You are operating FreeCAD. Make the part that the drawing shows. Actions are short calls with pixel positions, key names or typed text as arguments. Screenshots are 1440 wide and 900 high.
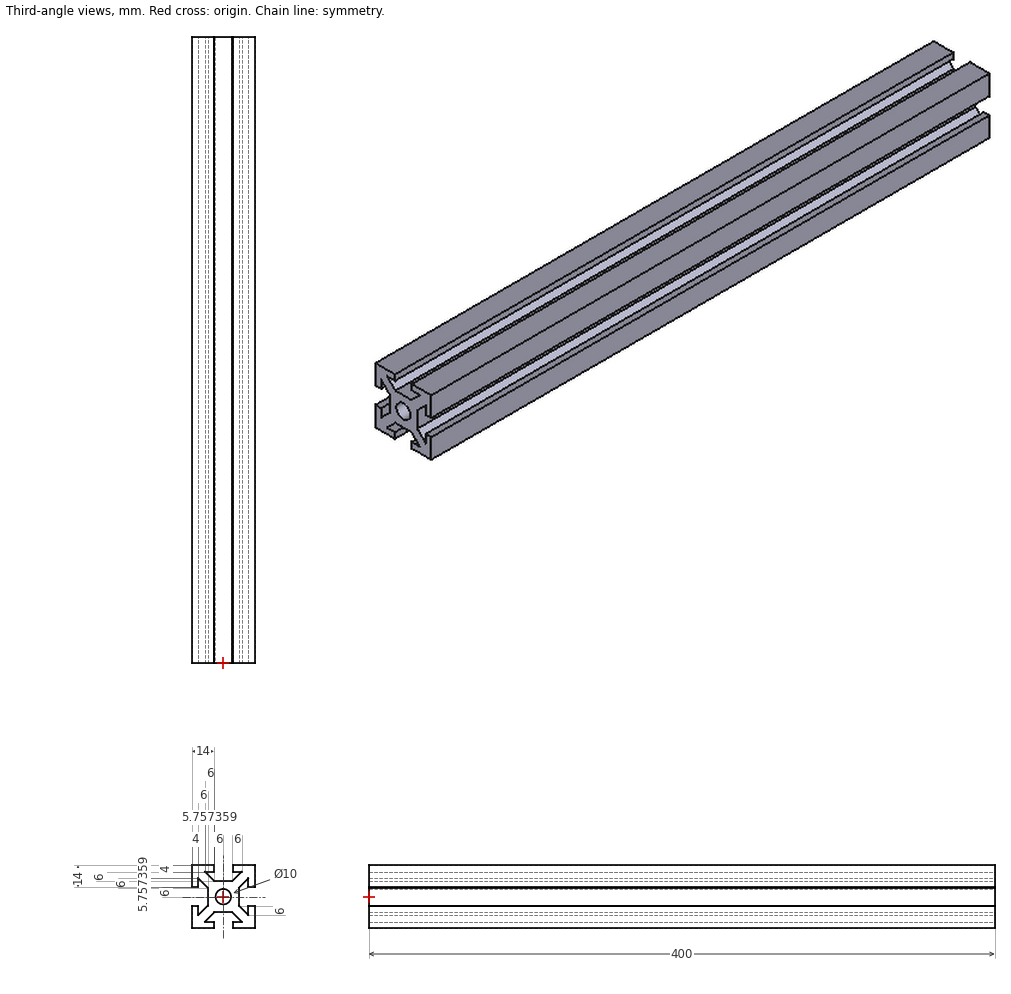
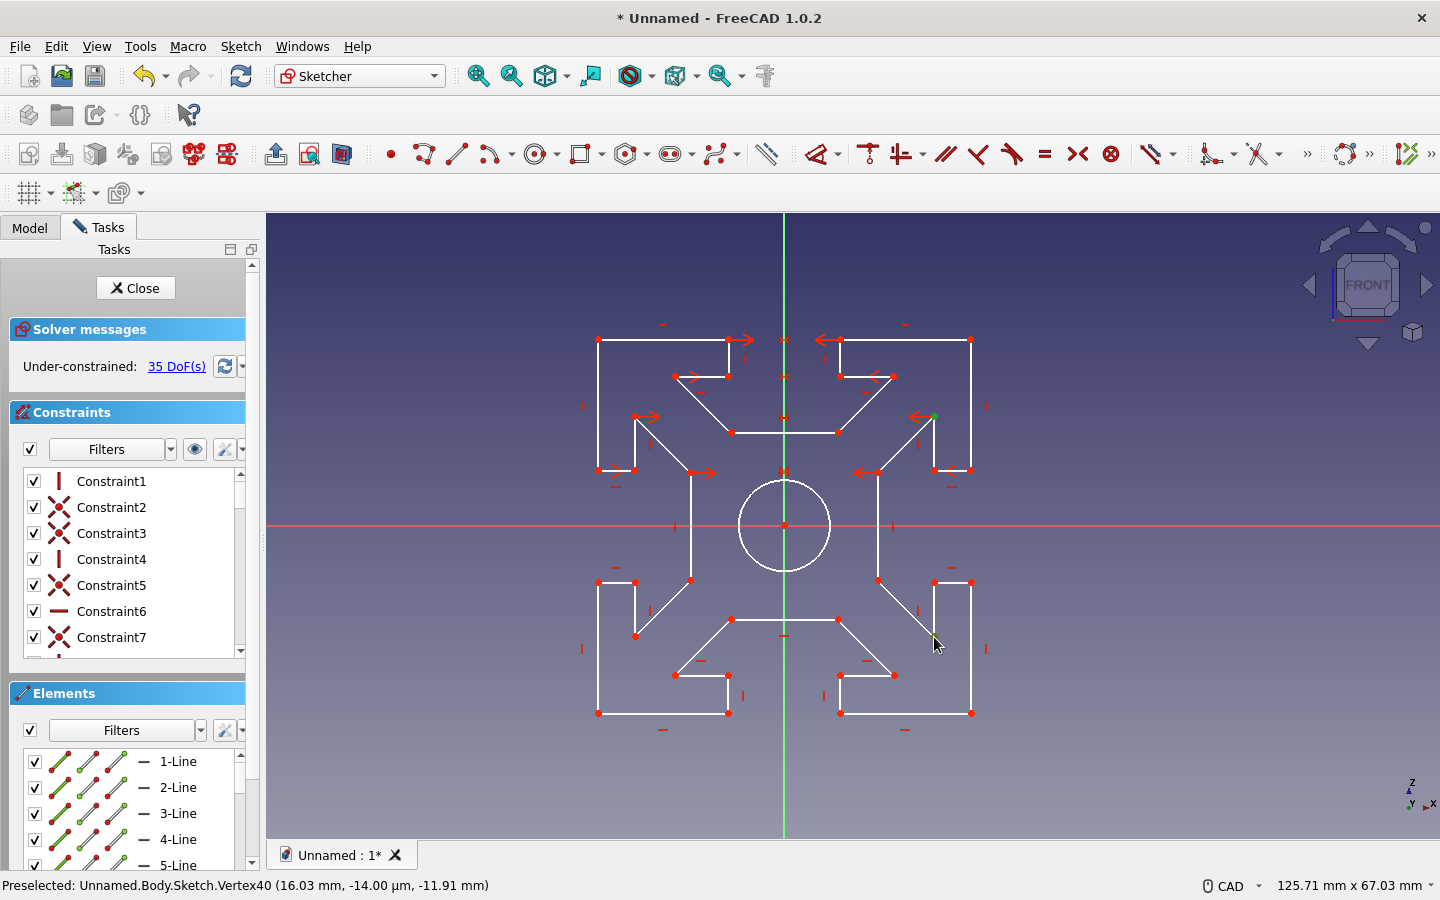
click(364, 526)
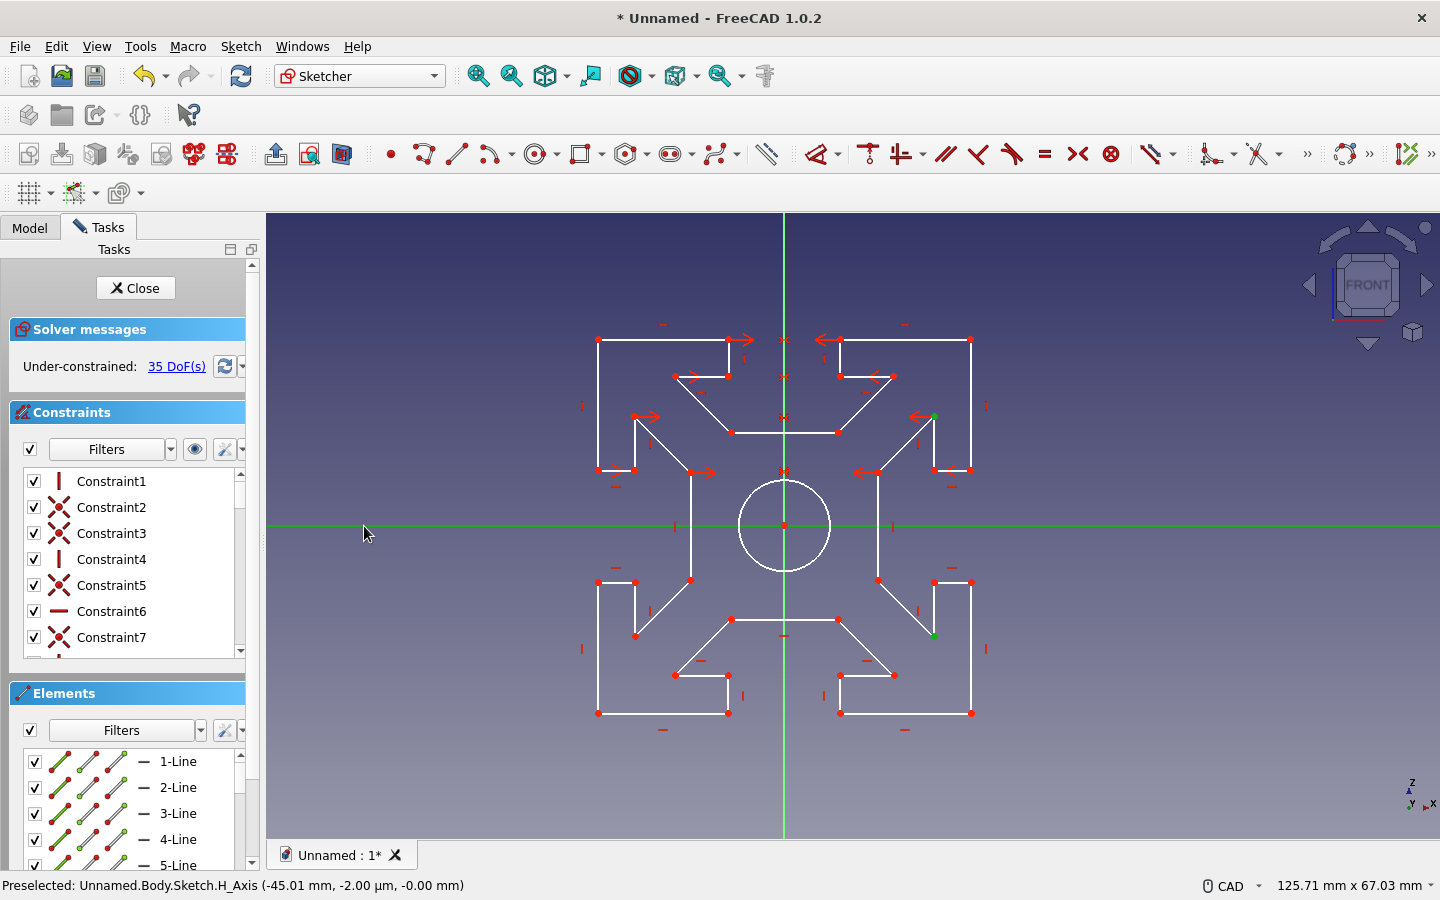
key(s)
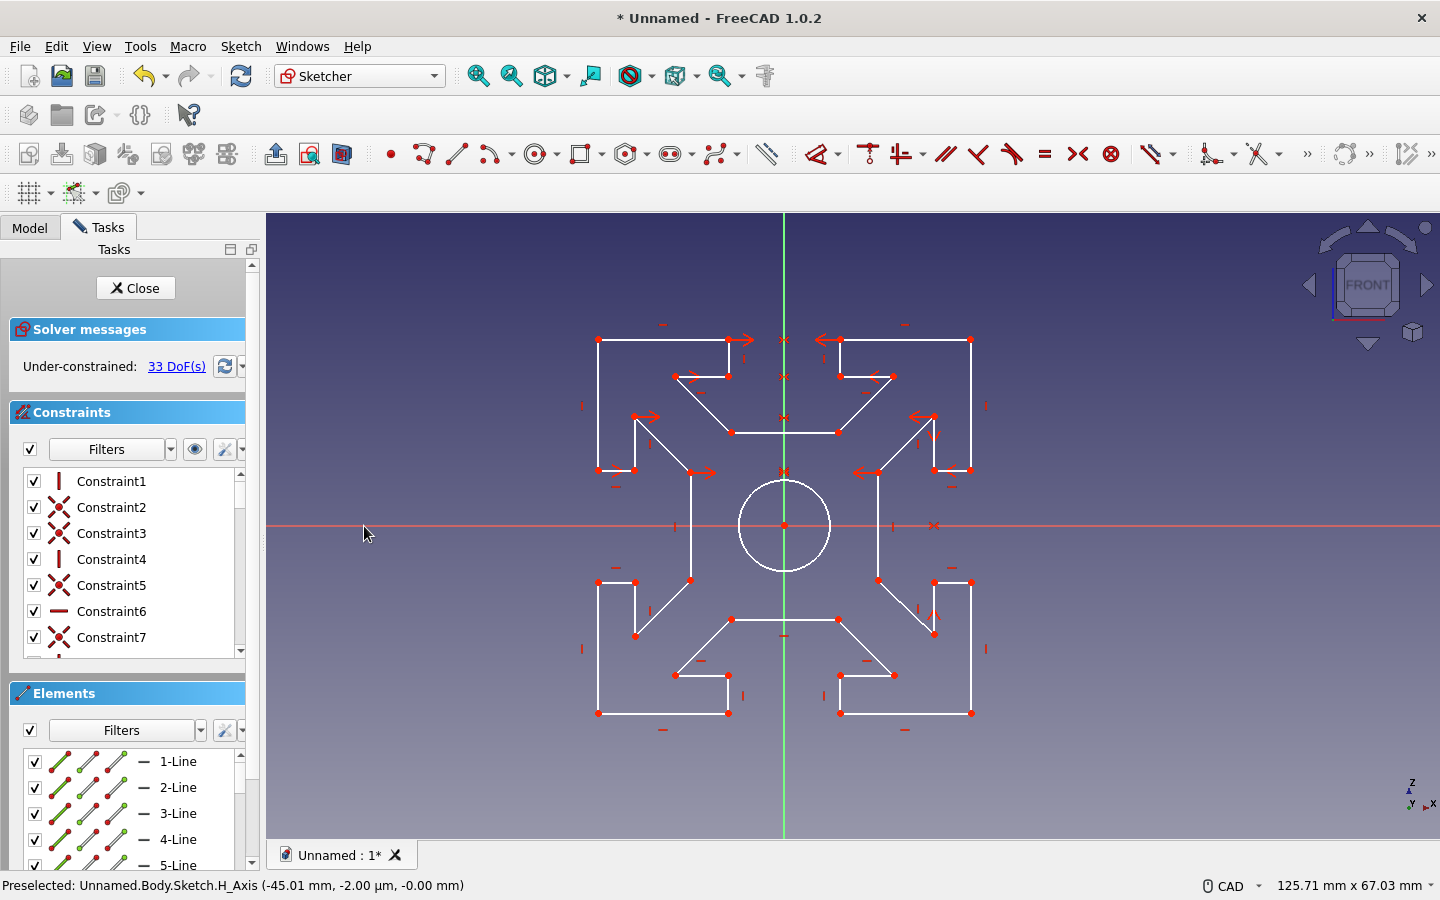
click(971, 471)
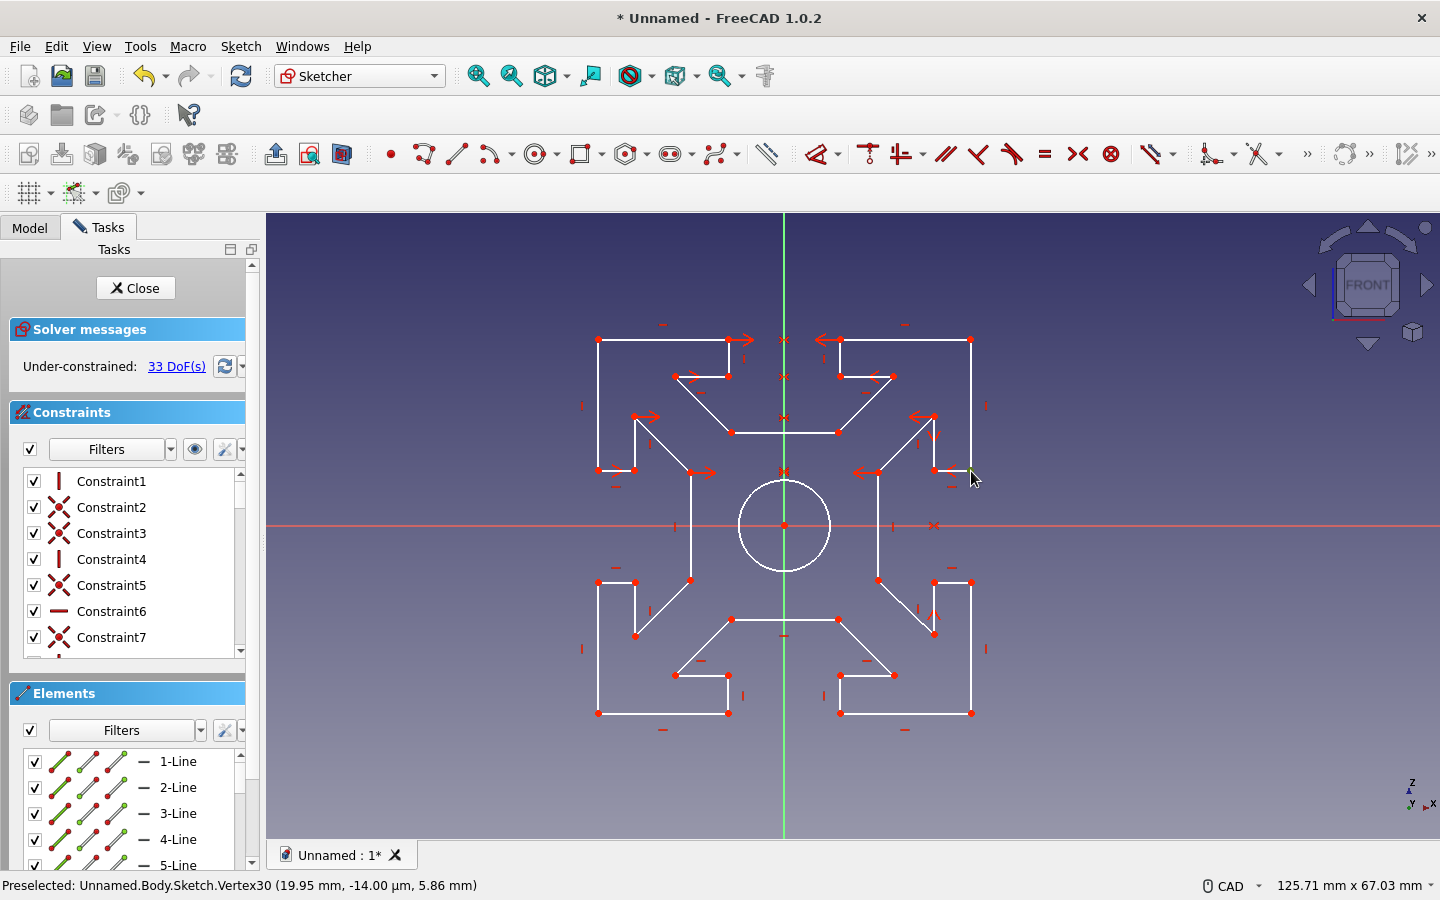
click(971, 583)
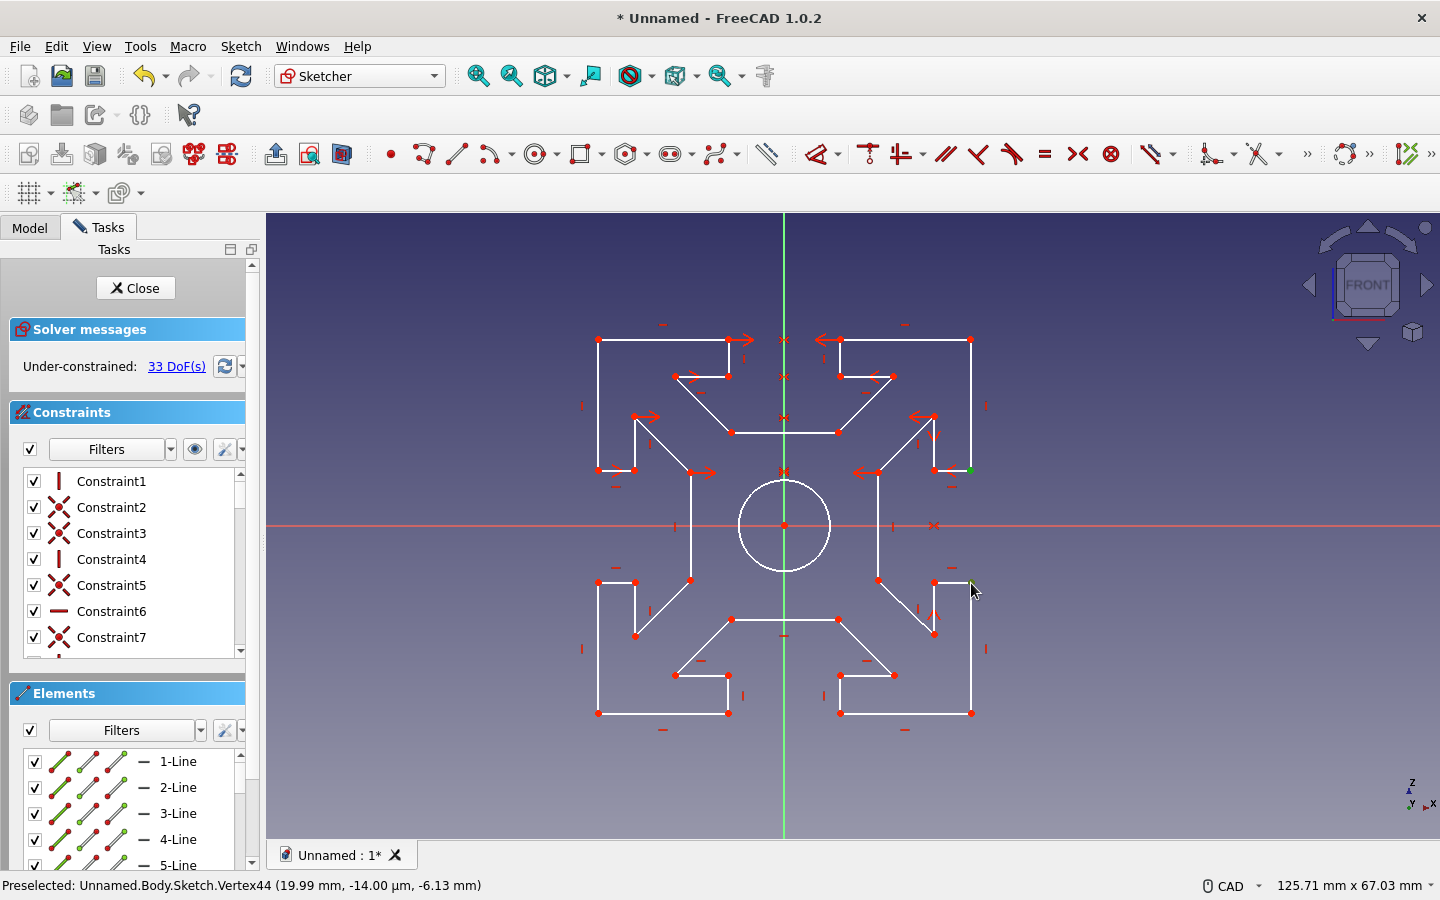
click(364, 526)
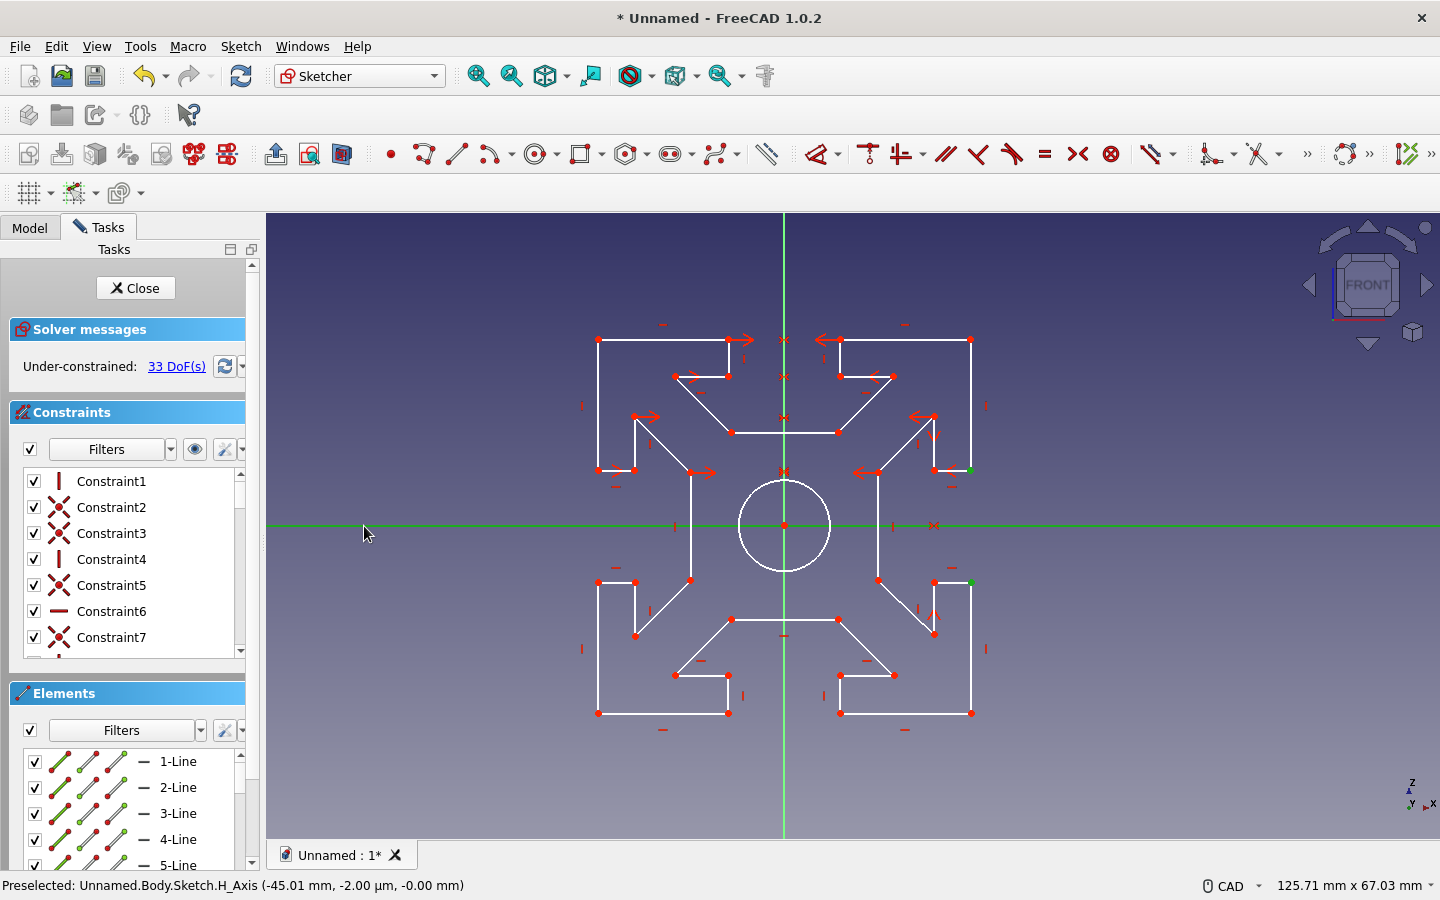
click(1078, 154)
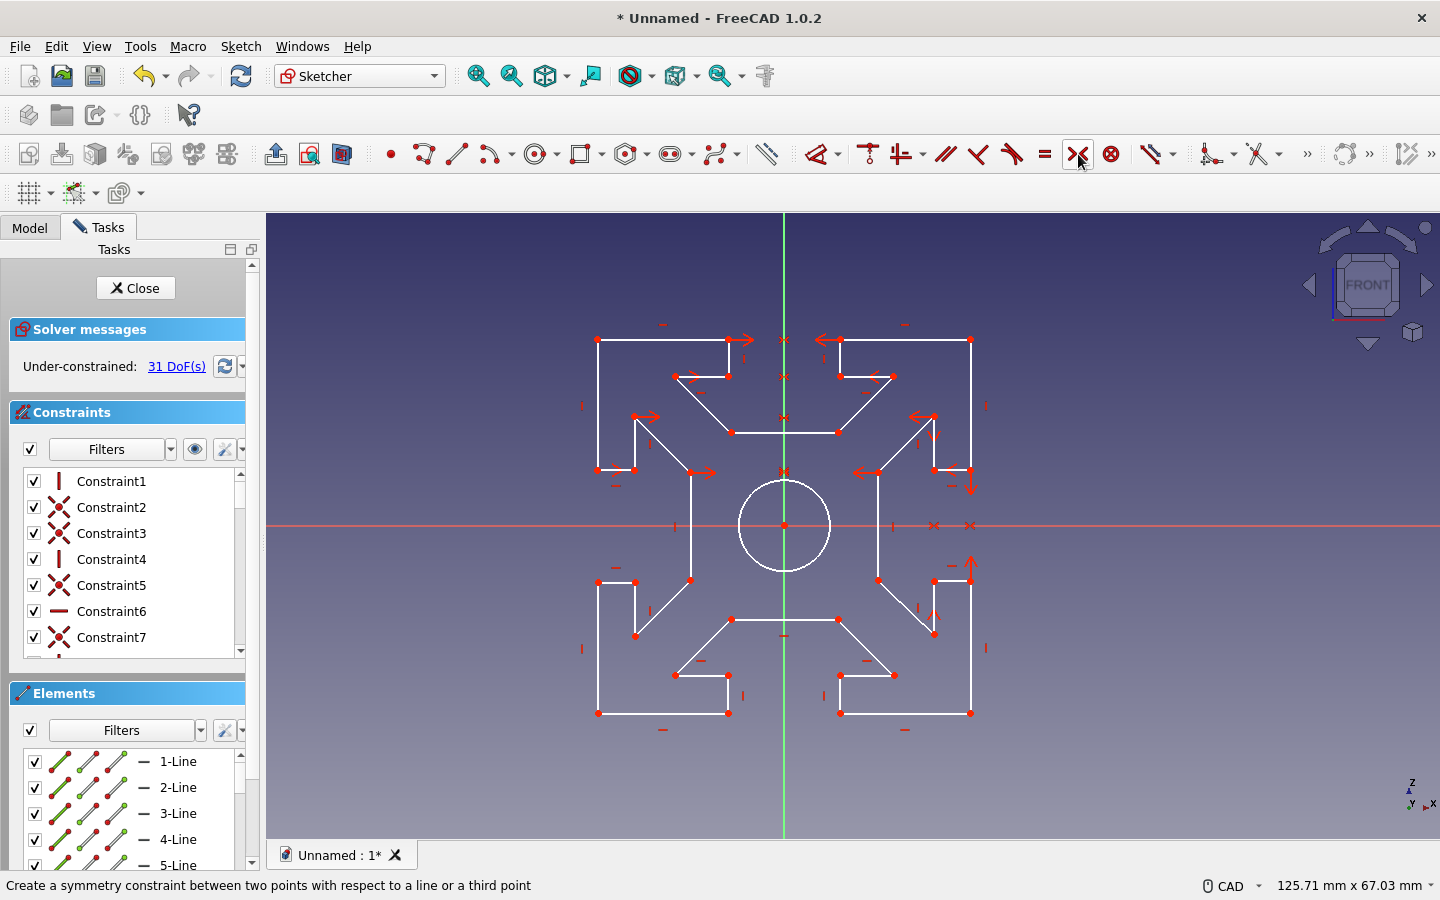
click(840, 340)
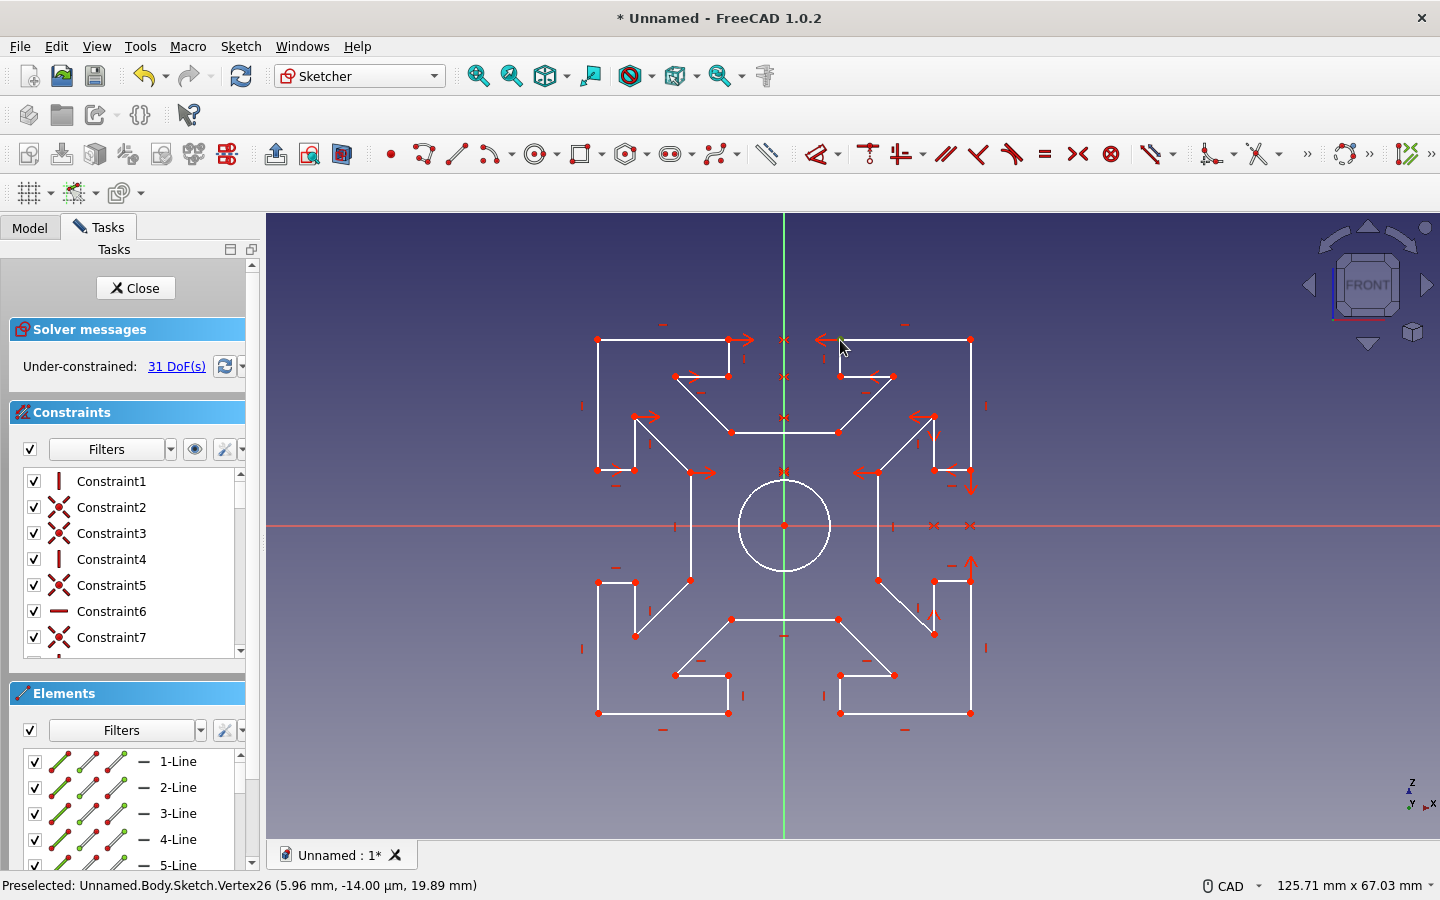
click(840, 714)